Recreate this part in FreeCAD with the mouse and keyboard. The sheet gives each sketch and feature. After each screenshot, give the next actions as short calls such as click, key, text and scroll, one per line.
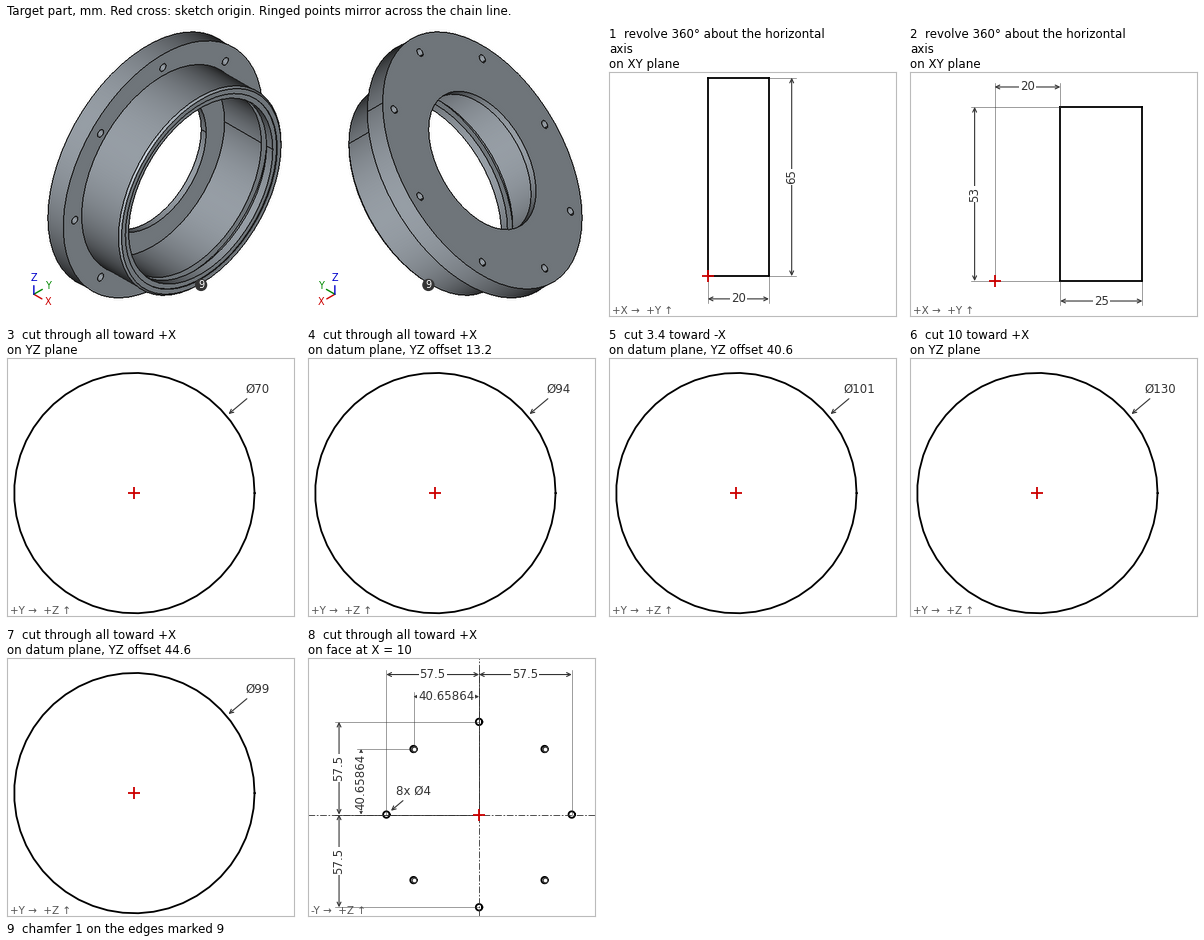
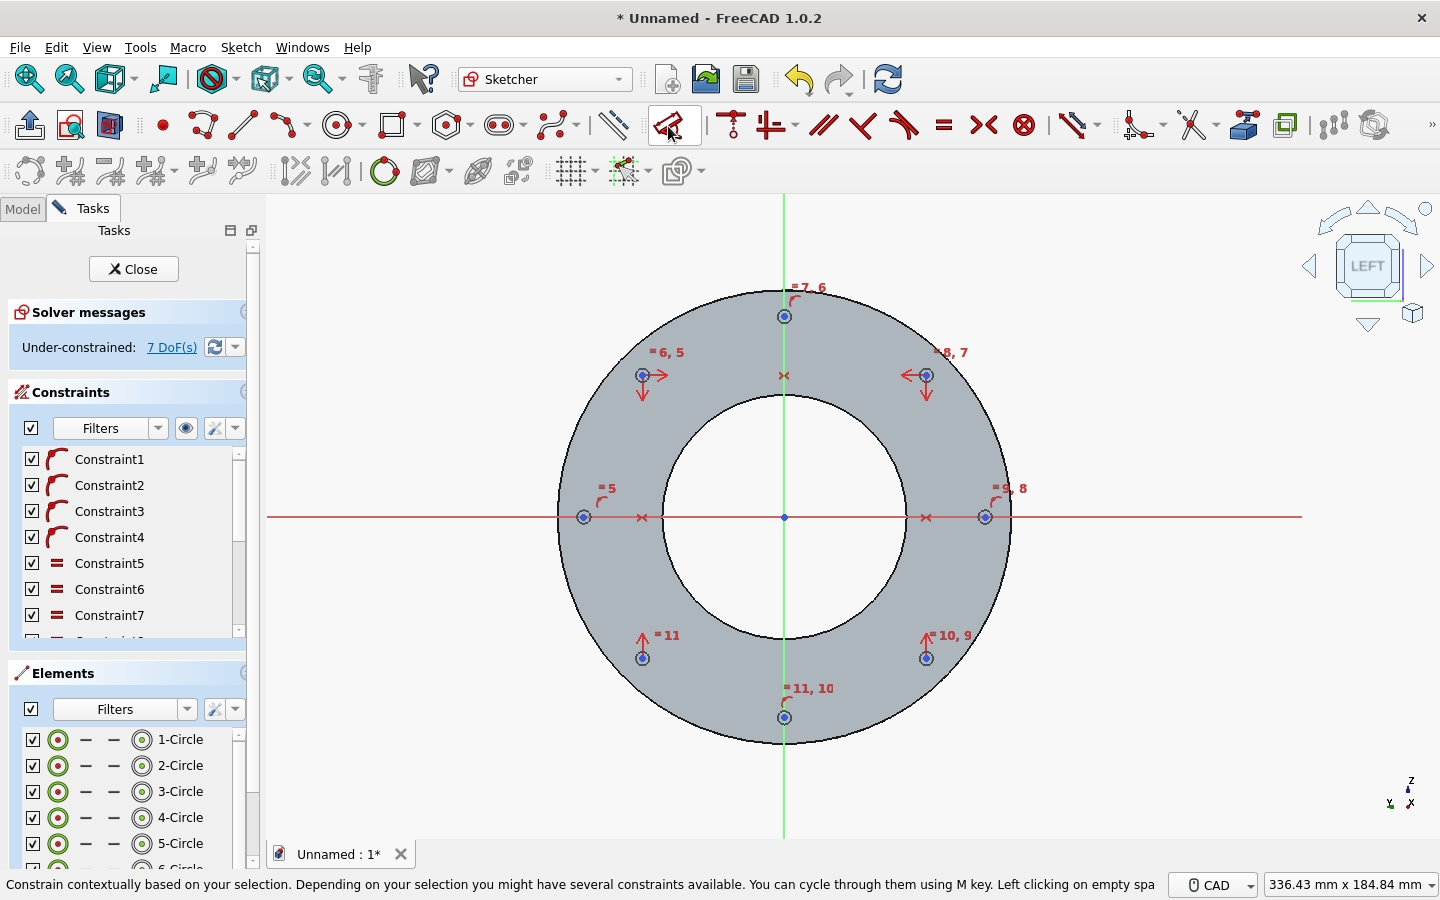
scroll(577, 517, up, 6)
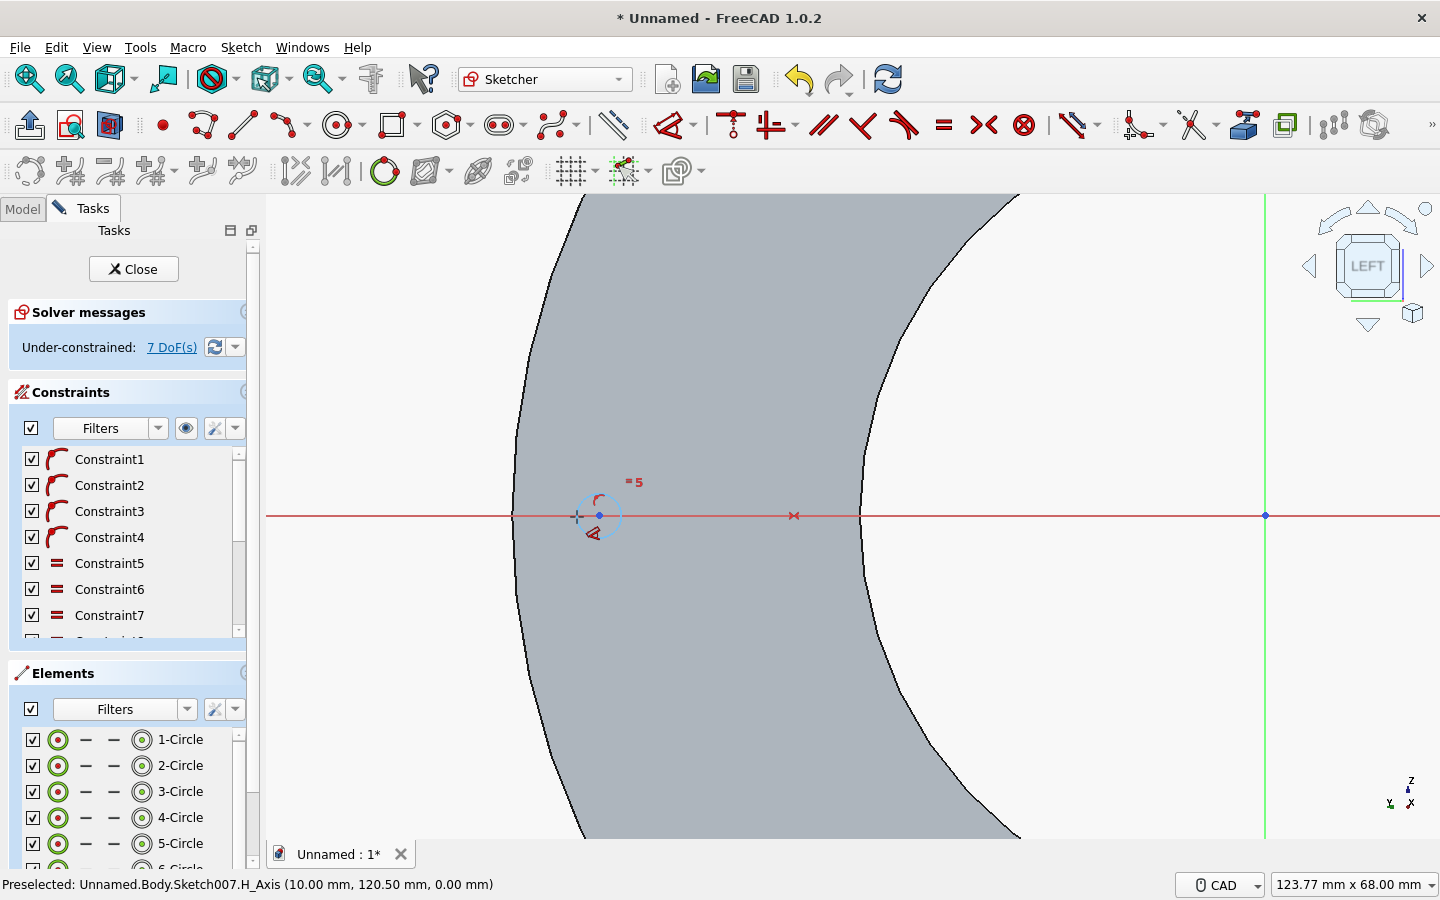
click(577, 515)
click(553, 488)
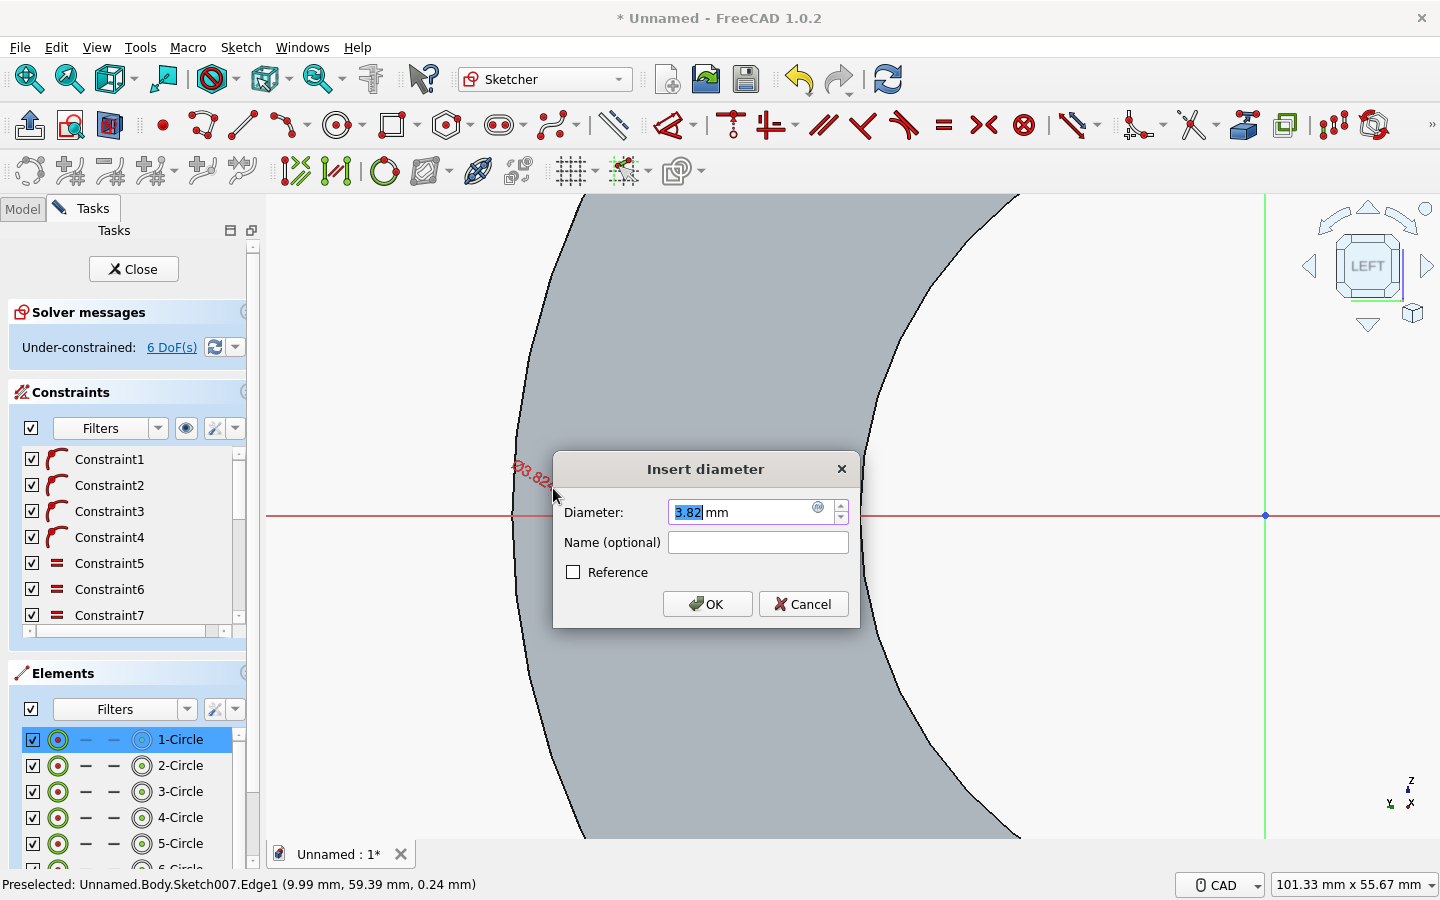
text(4)
key(Return)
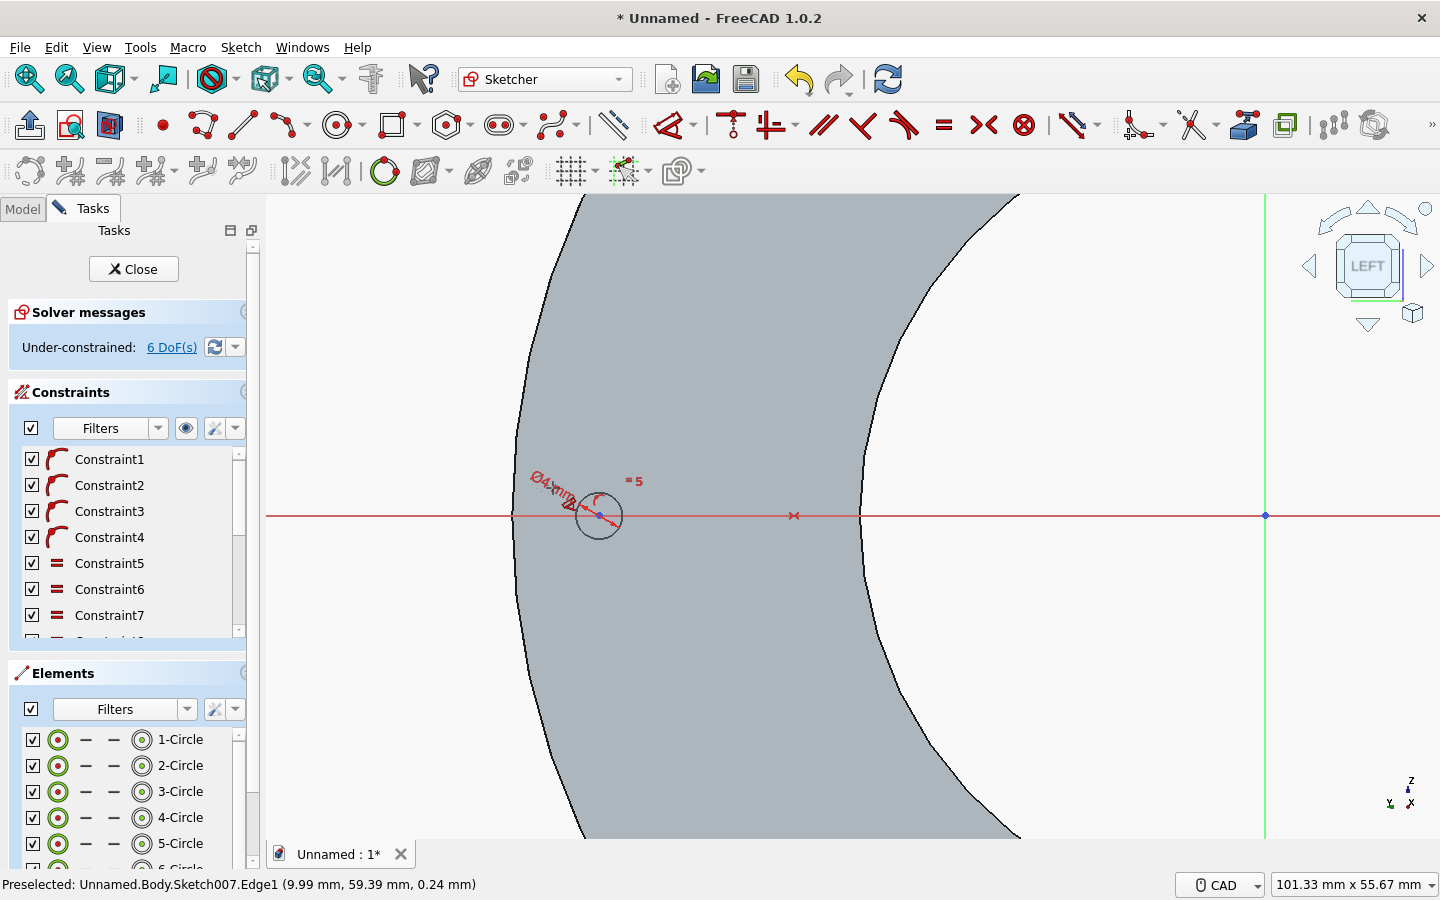
click(599, 516)
click(932, 550)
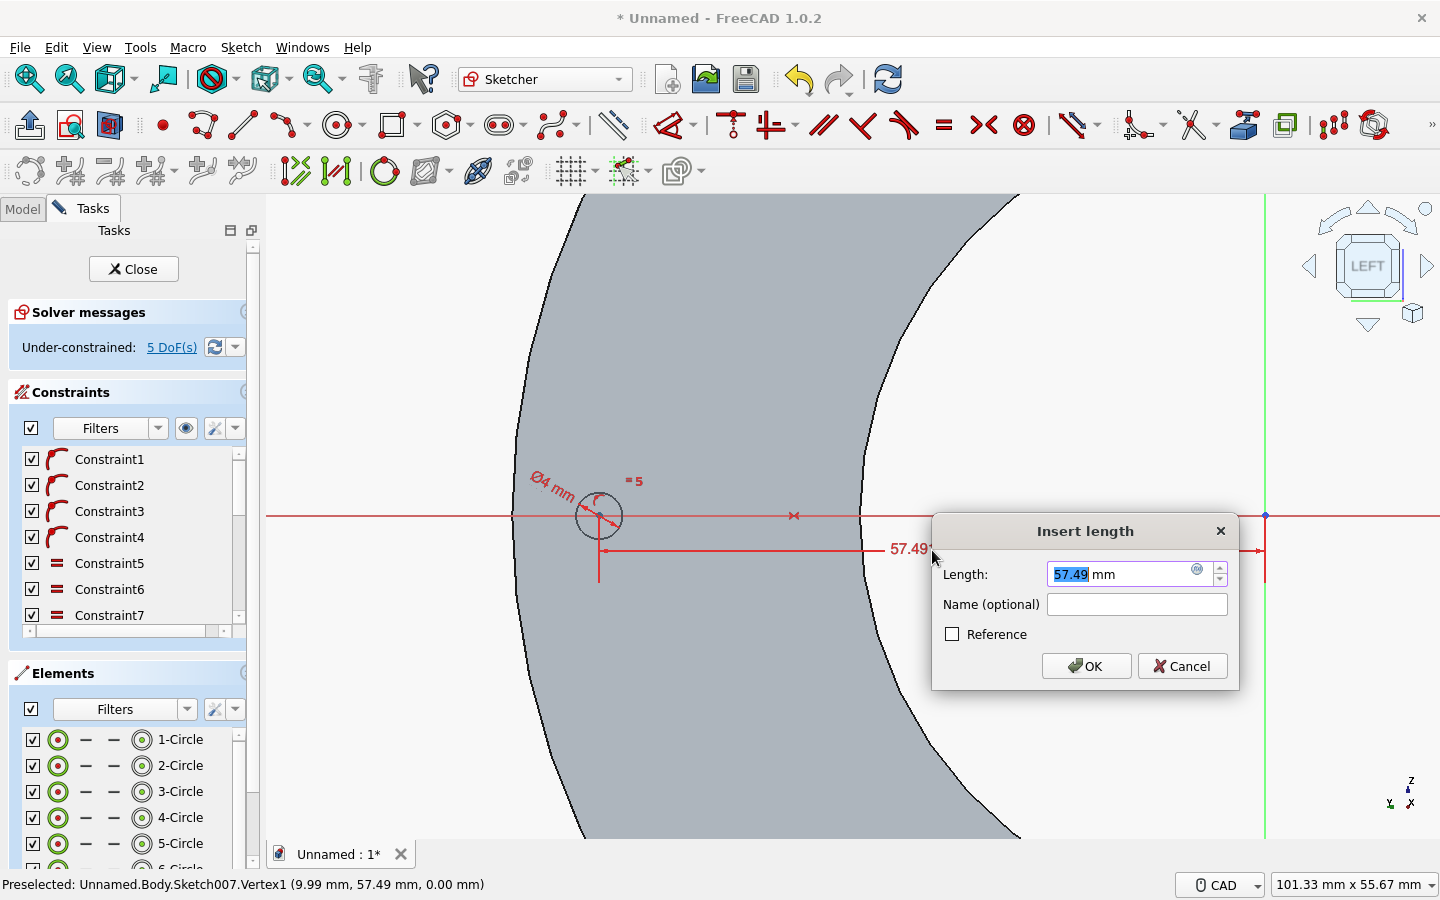
text(57.5)
key(Return)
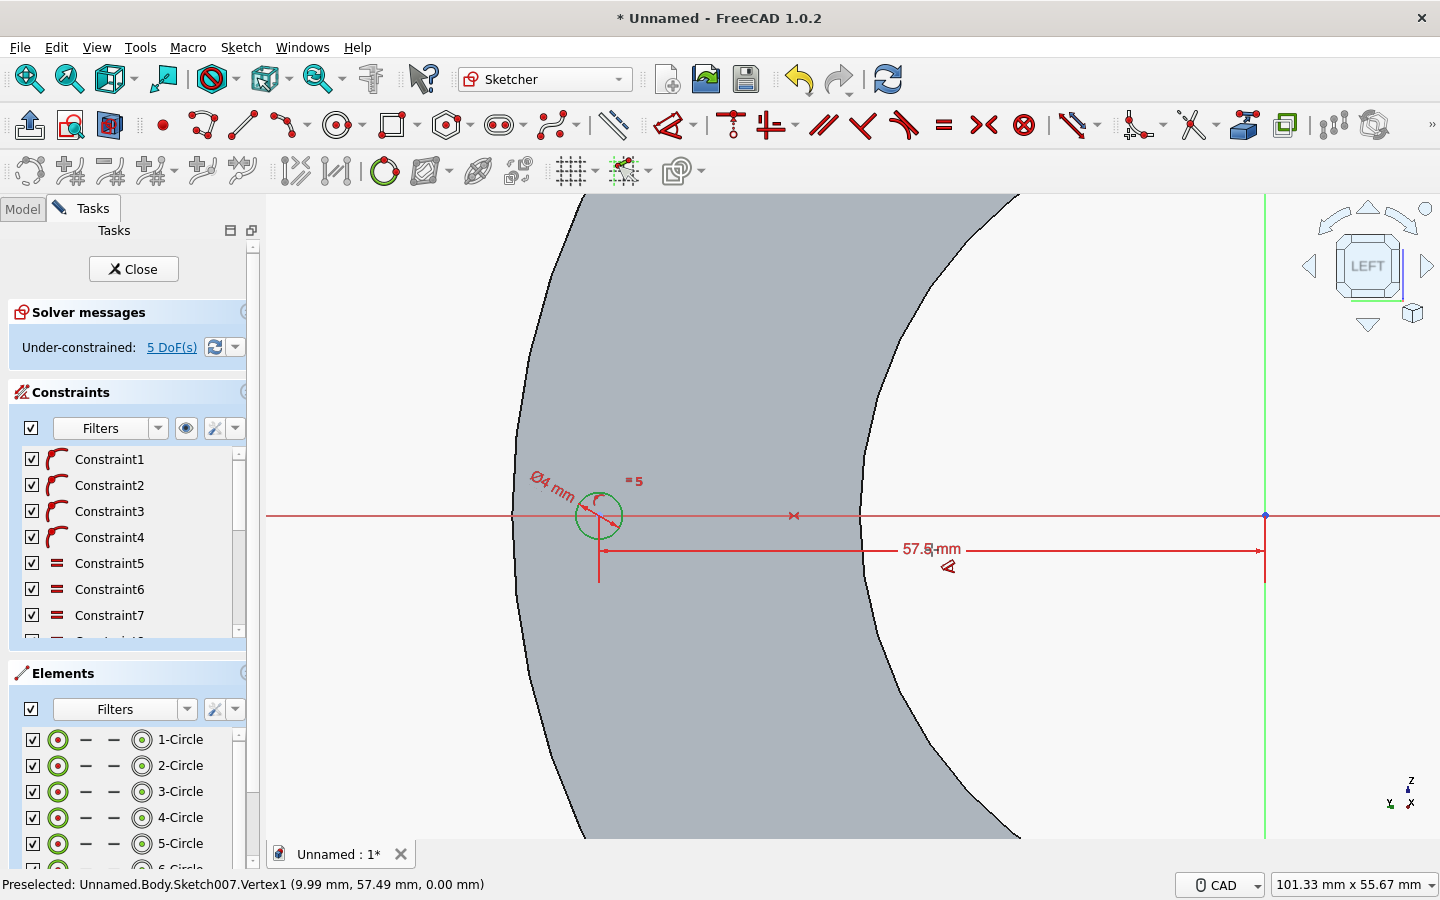
scroll(577, 517, down, 6)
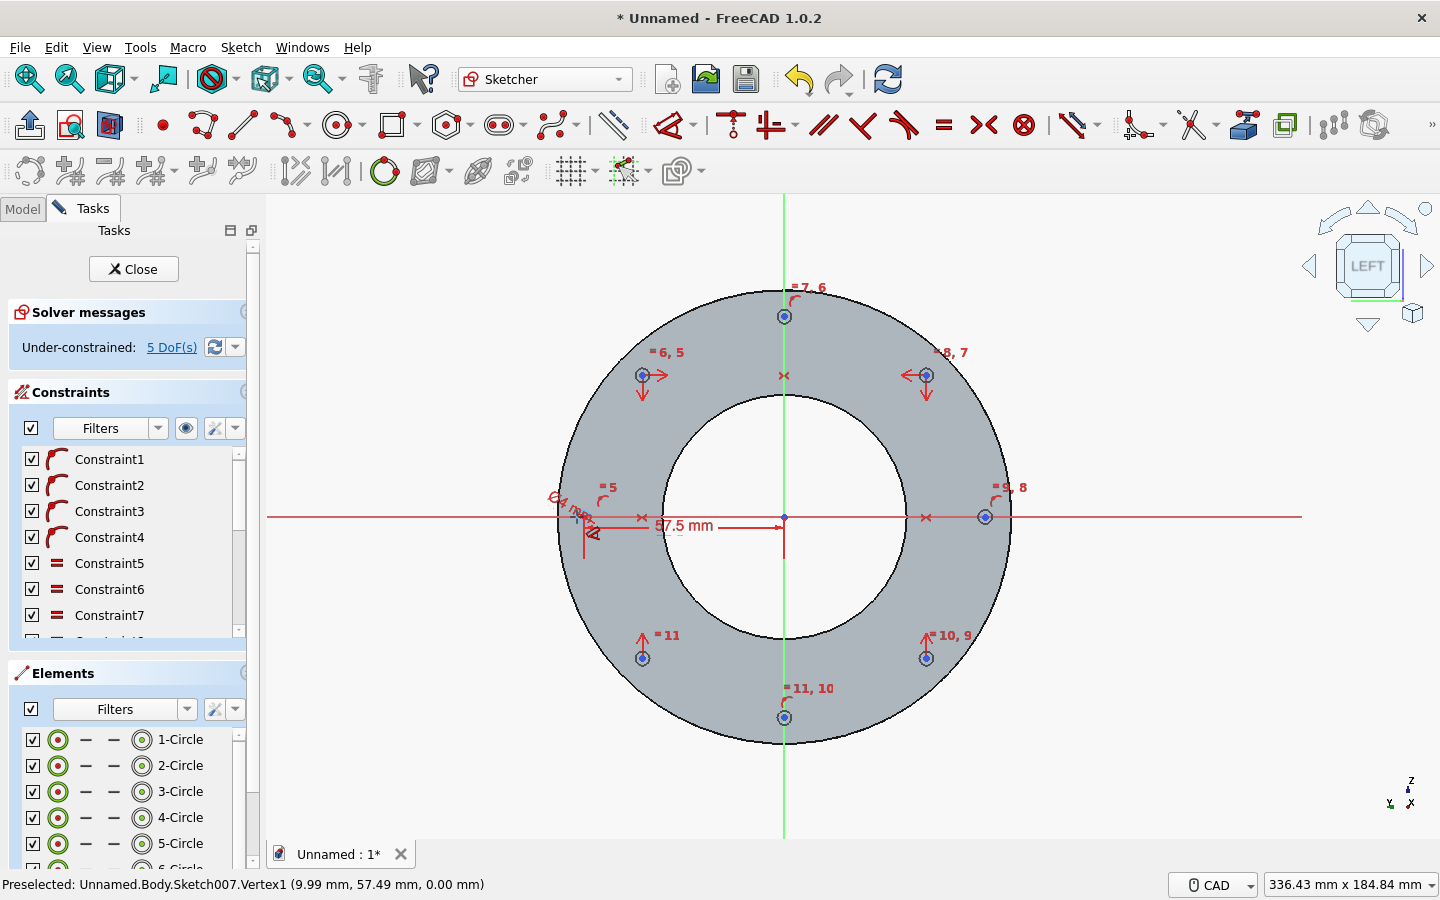
click(784, 317)
click(818, 417)